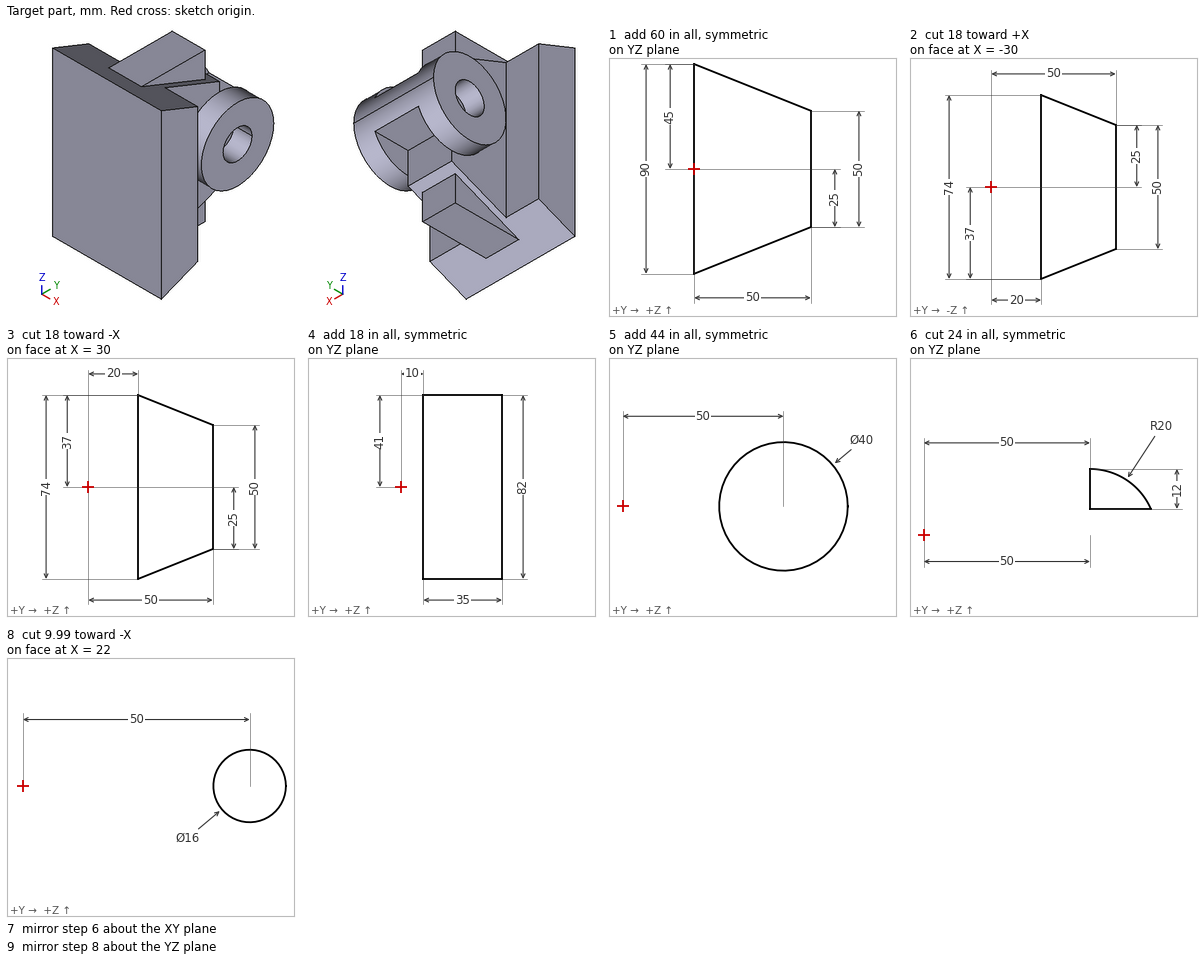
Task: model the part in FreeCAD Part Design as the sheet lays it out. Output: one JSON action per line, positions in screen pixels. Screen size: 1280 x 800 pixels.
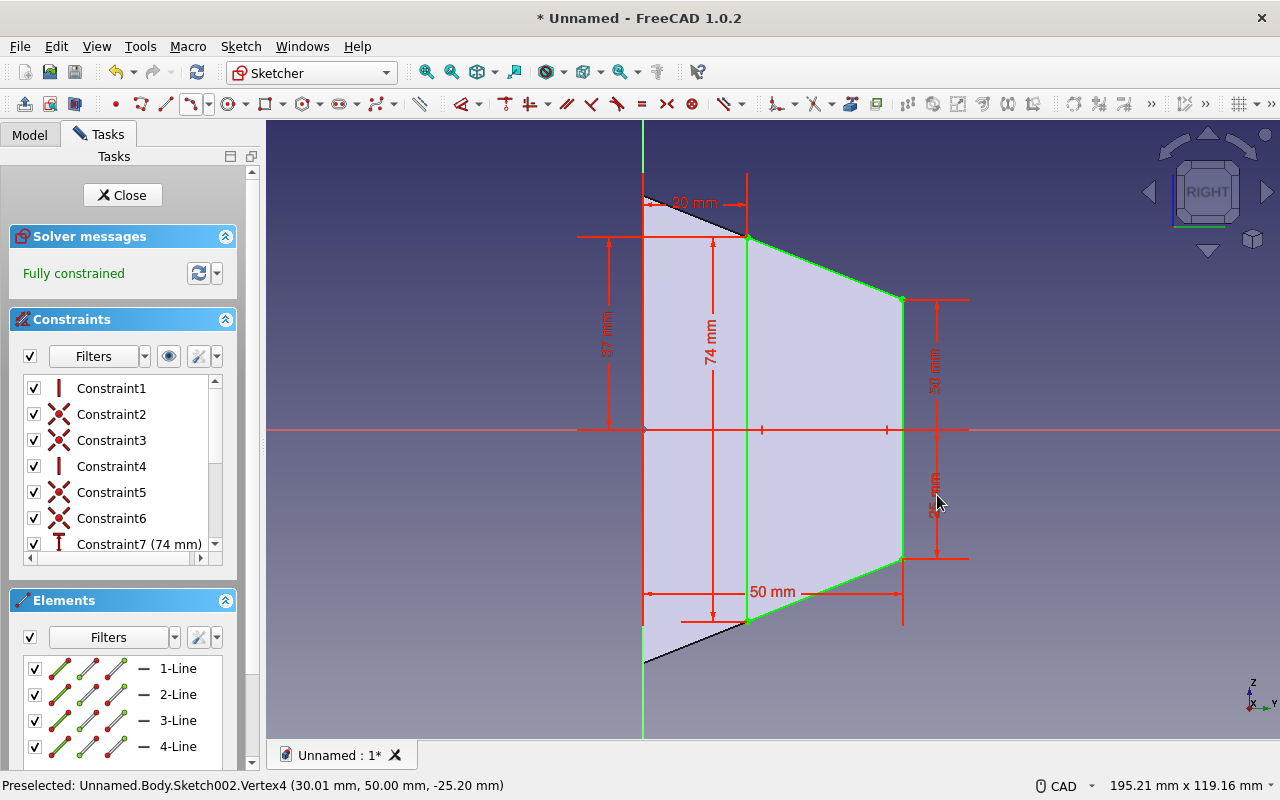
{"action": "left_click", "coordinate": [123, 195]}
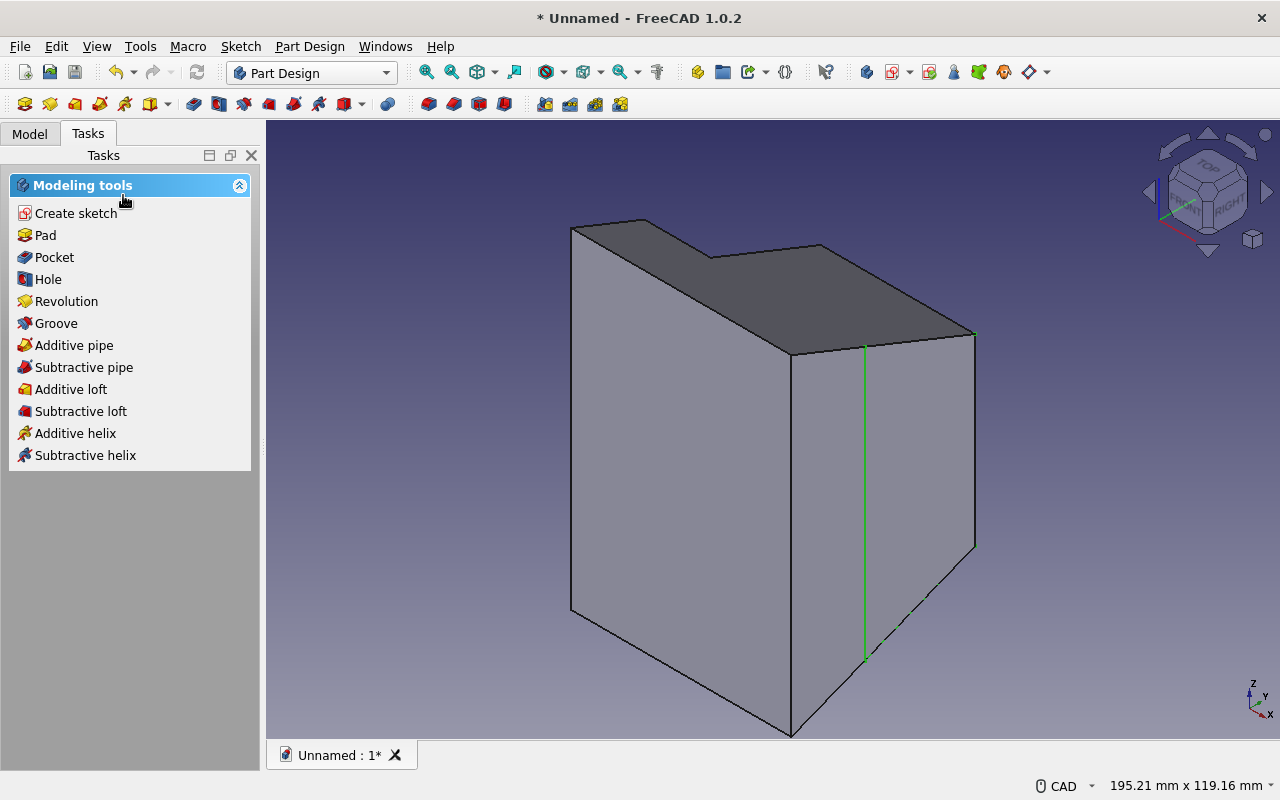
{"action": "left_click", "coordinate": [194, 104]}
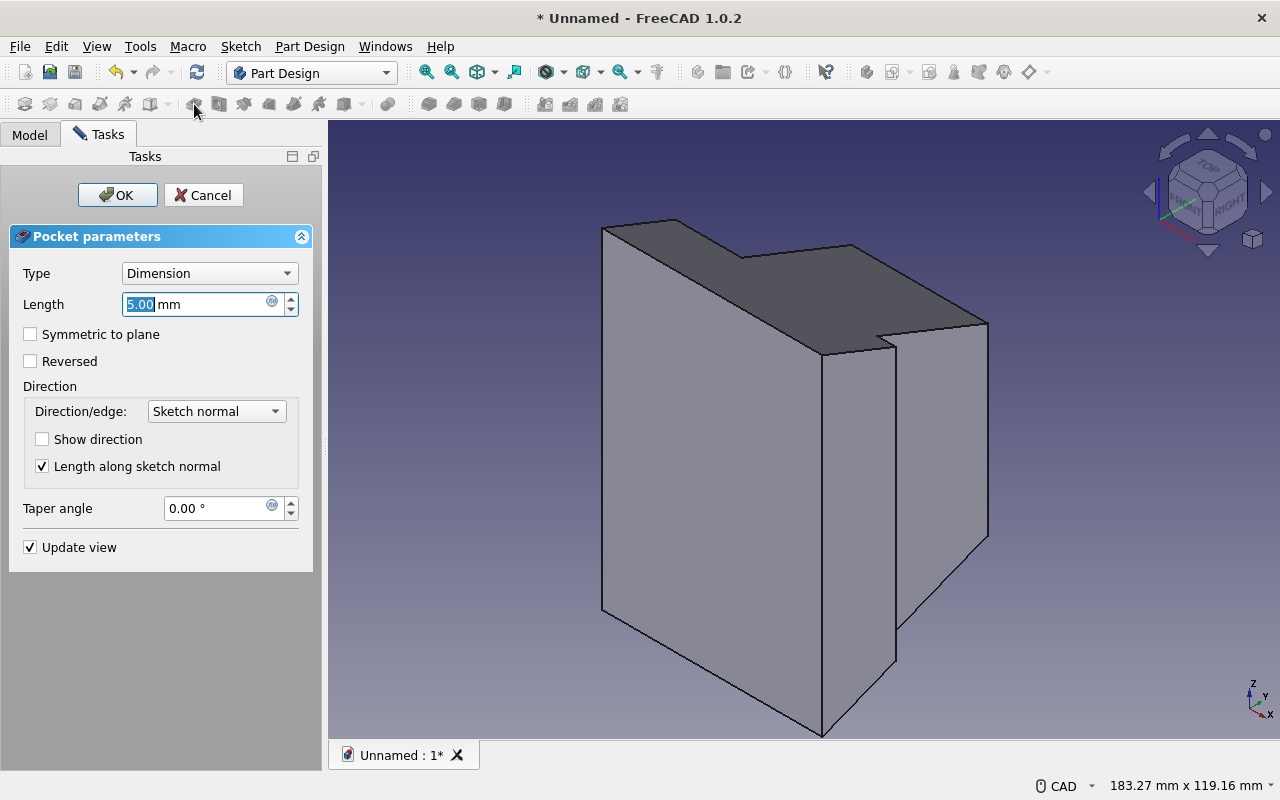
{"action": "type", "text": "18"}
{"action": "key", "text": "Tab"}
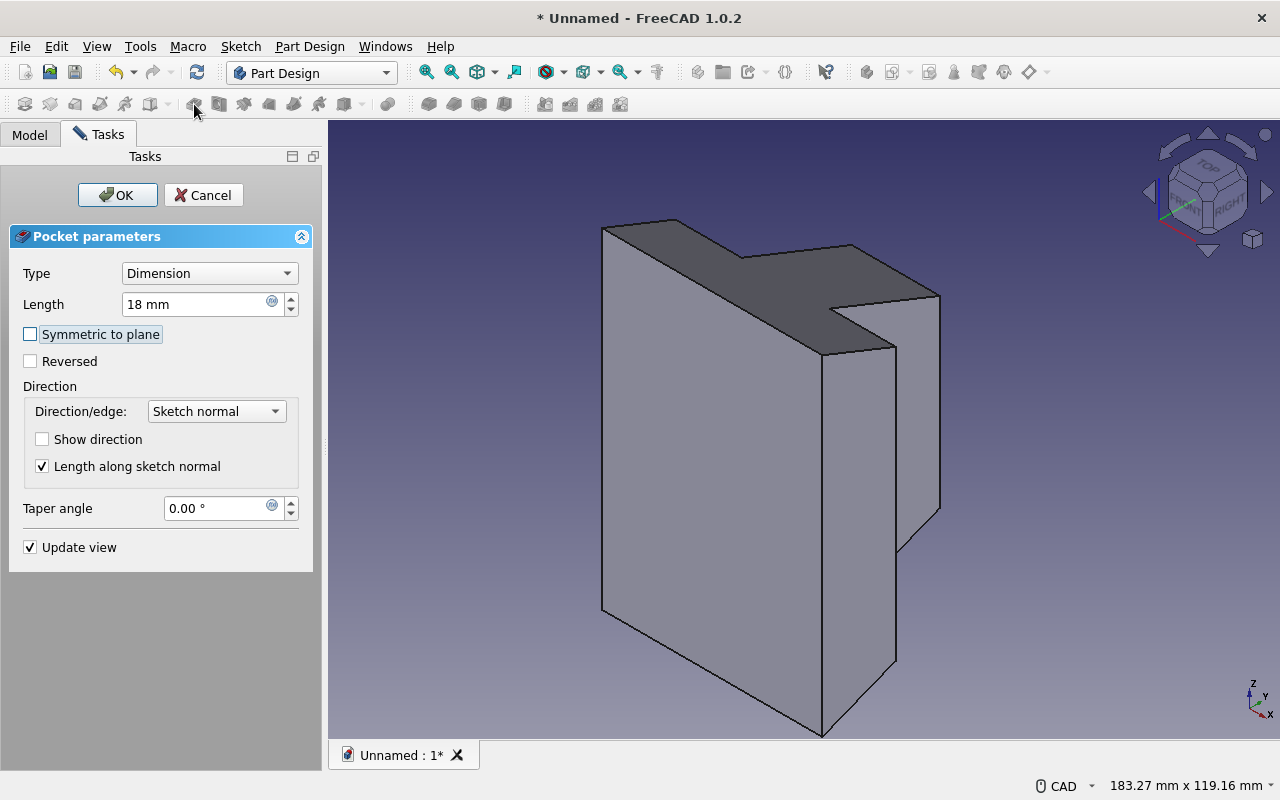
{"action": "left_click", "coordinate": [118, 195]}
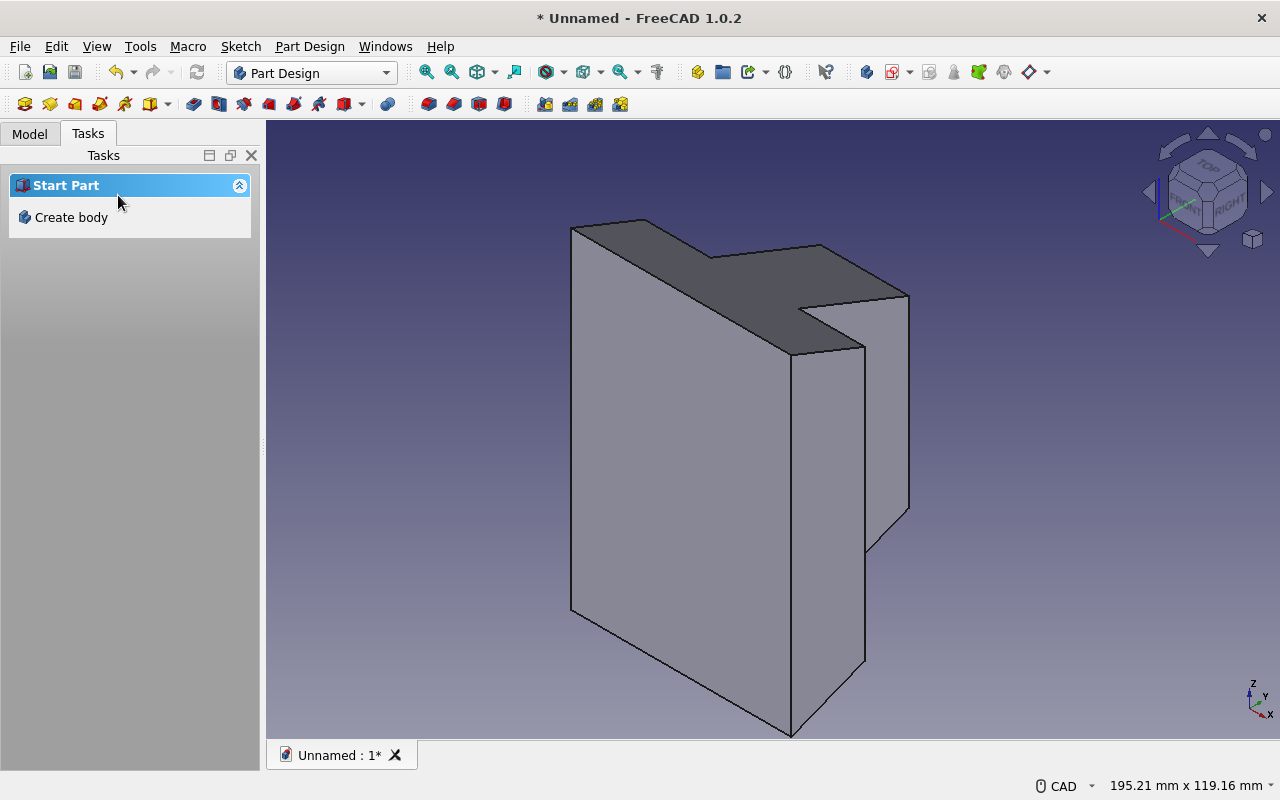
{"action": "left_click", "coordinate": [892, 72]}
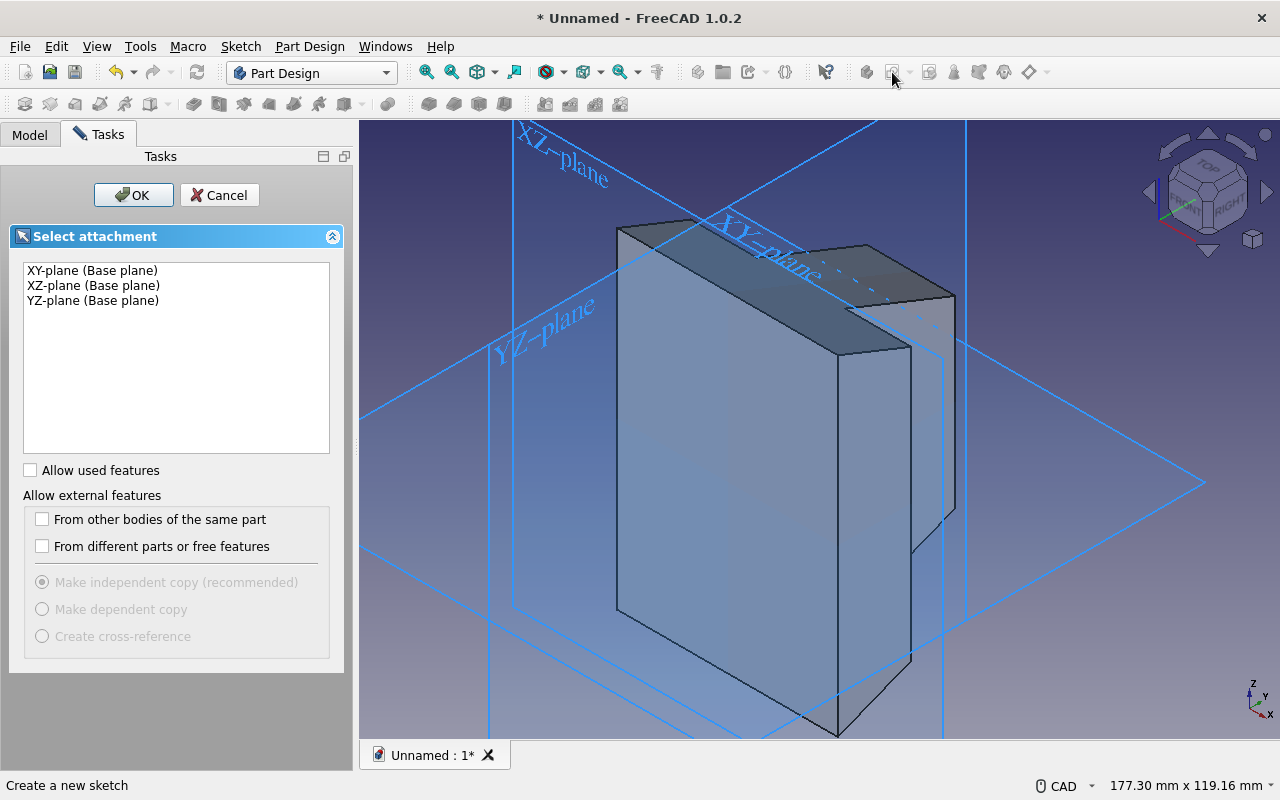
{"action": "left_click", "coordinate": [84, 300]}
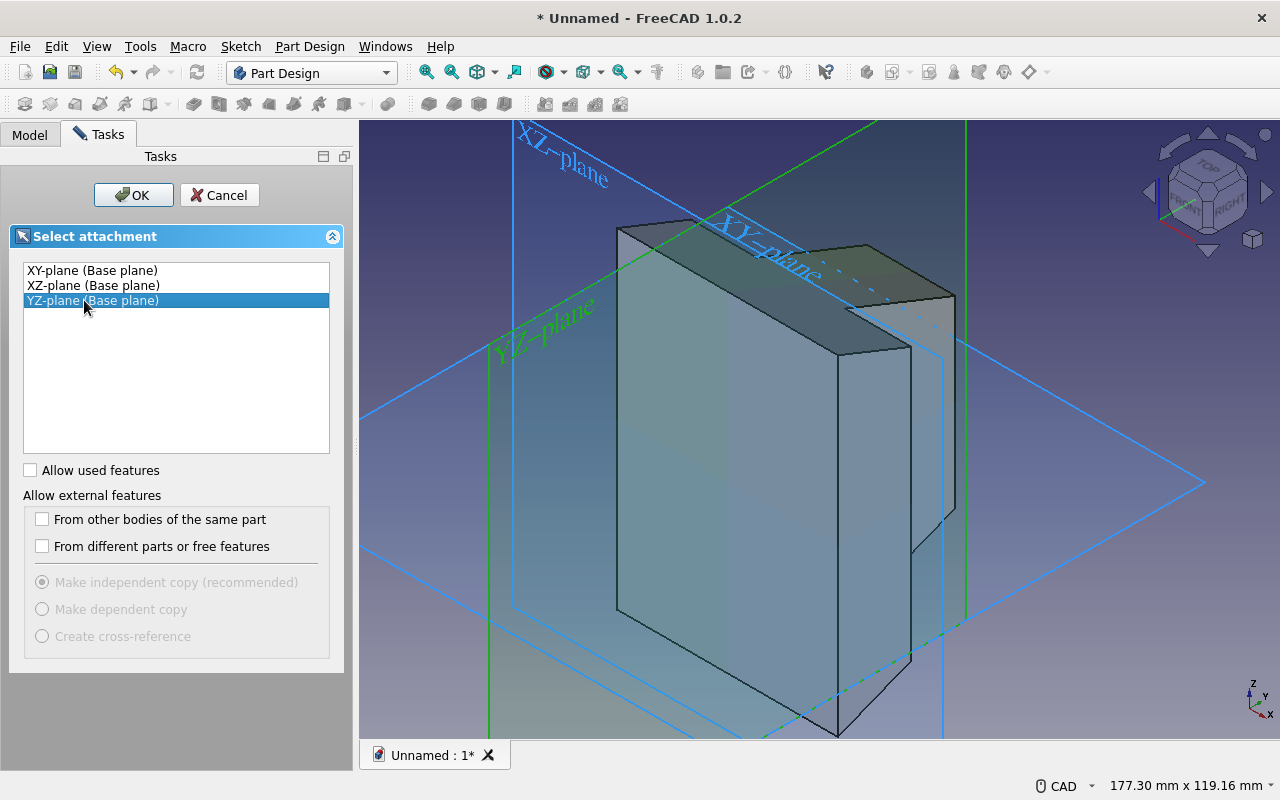
{"action": "left_click", "coordinate": [134, 195]}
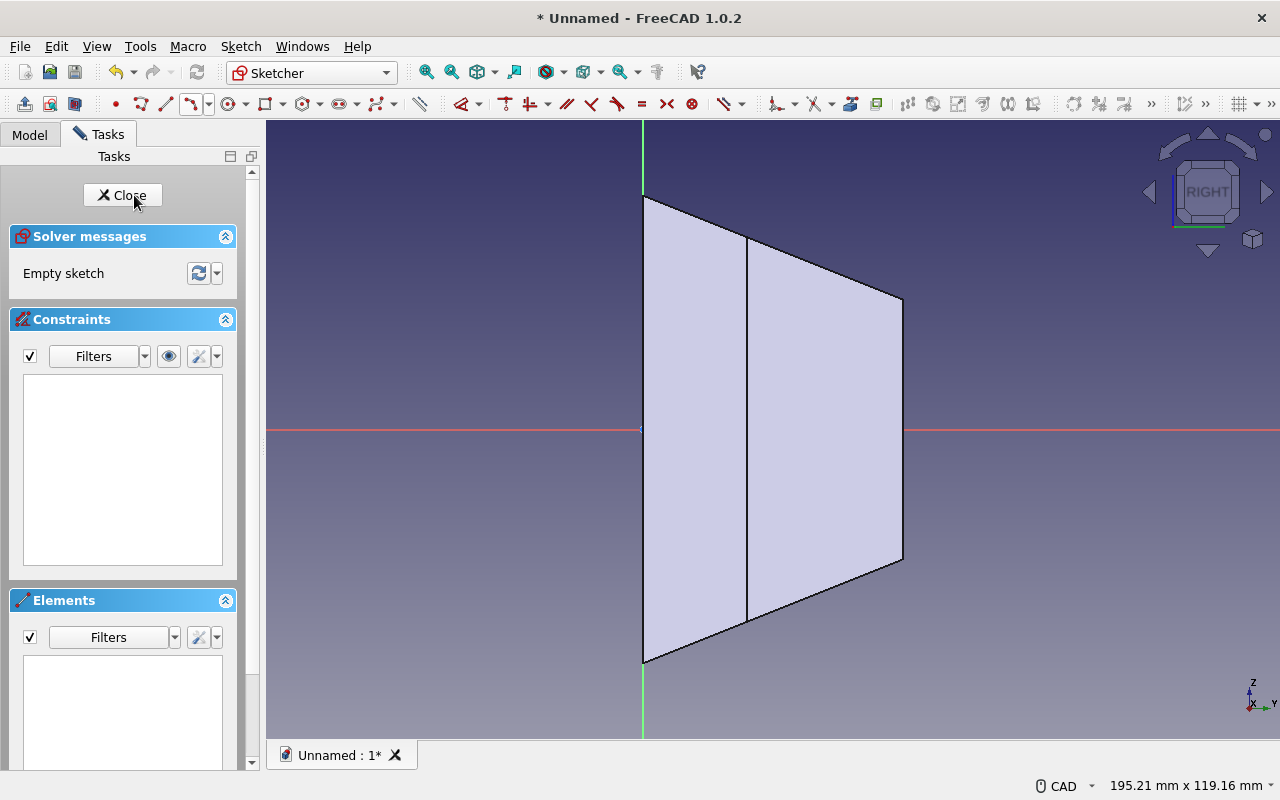
{"action": "left_click", "coordinate": [75, 104]}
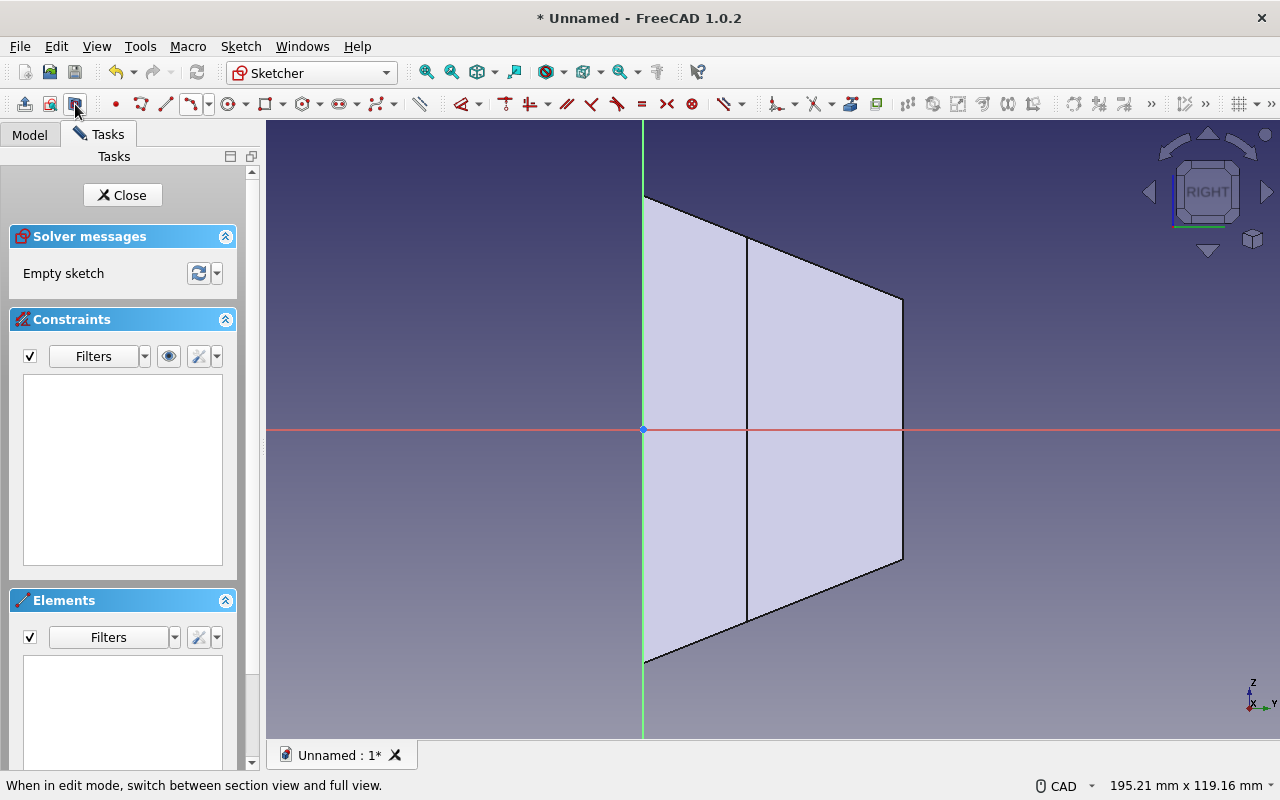
{"action": "key", "text": "g r"}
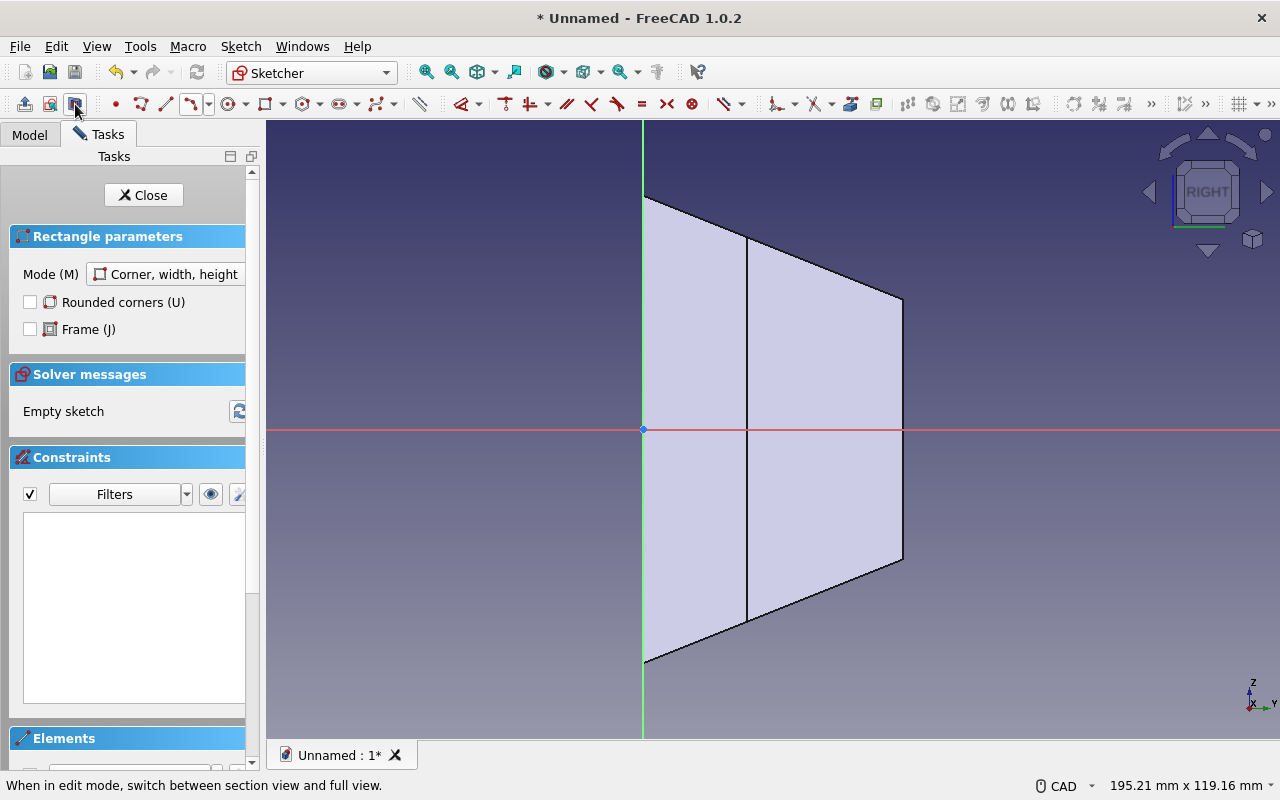
{"action": "left_click", "coordinate": [695, 217]}
{"action": "mouse_move", "coordinate": [877, 642]}